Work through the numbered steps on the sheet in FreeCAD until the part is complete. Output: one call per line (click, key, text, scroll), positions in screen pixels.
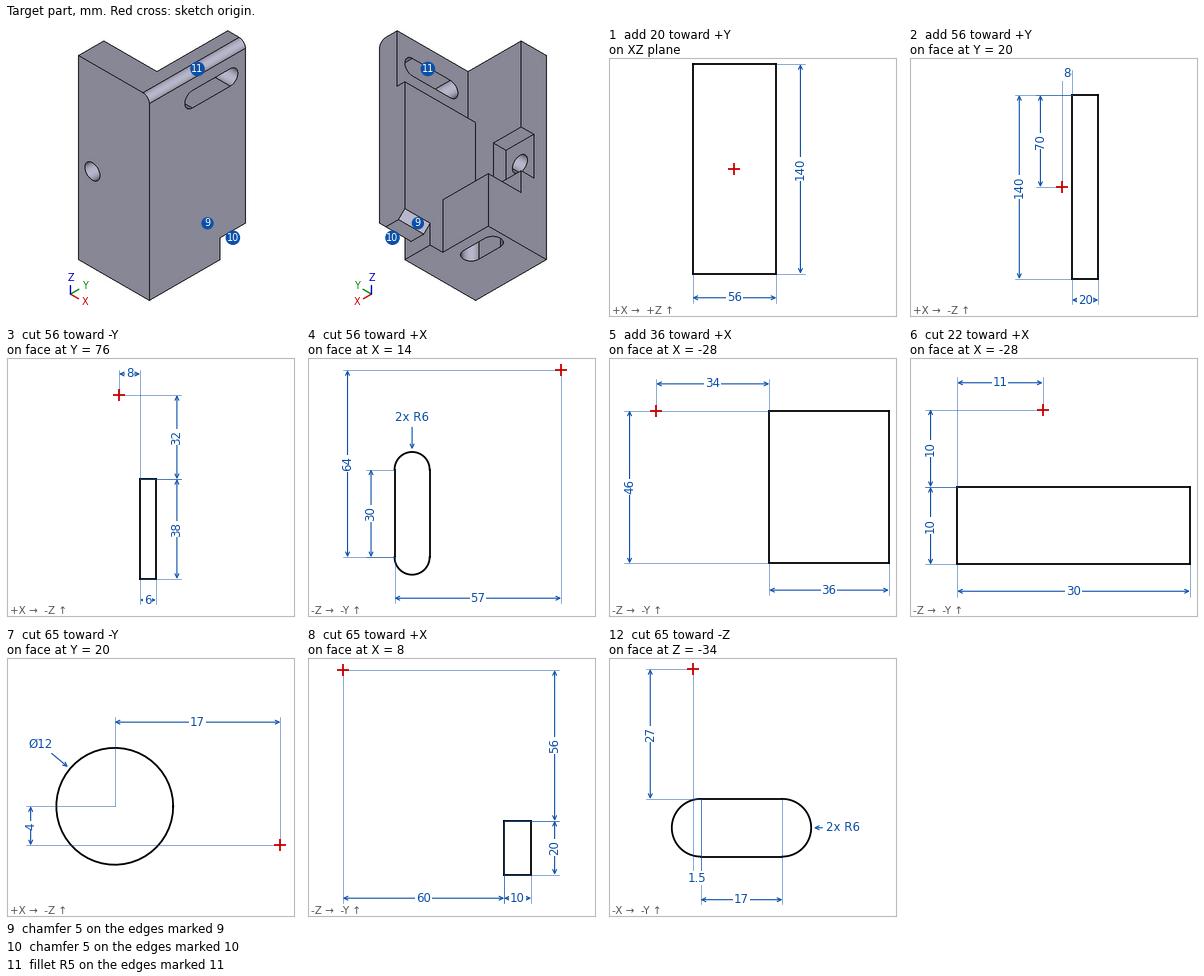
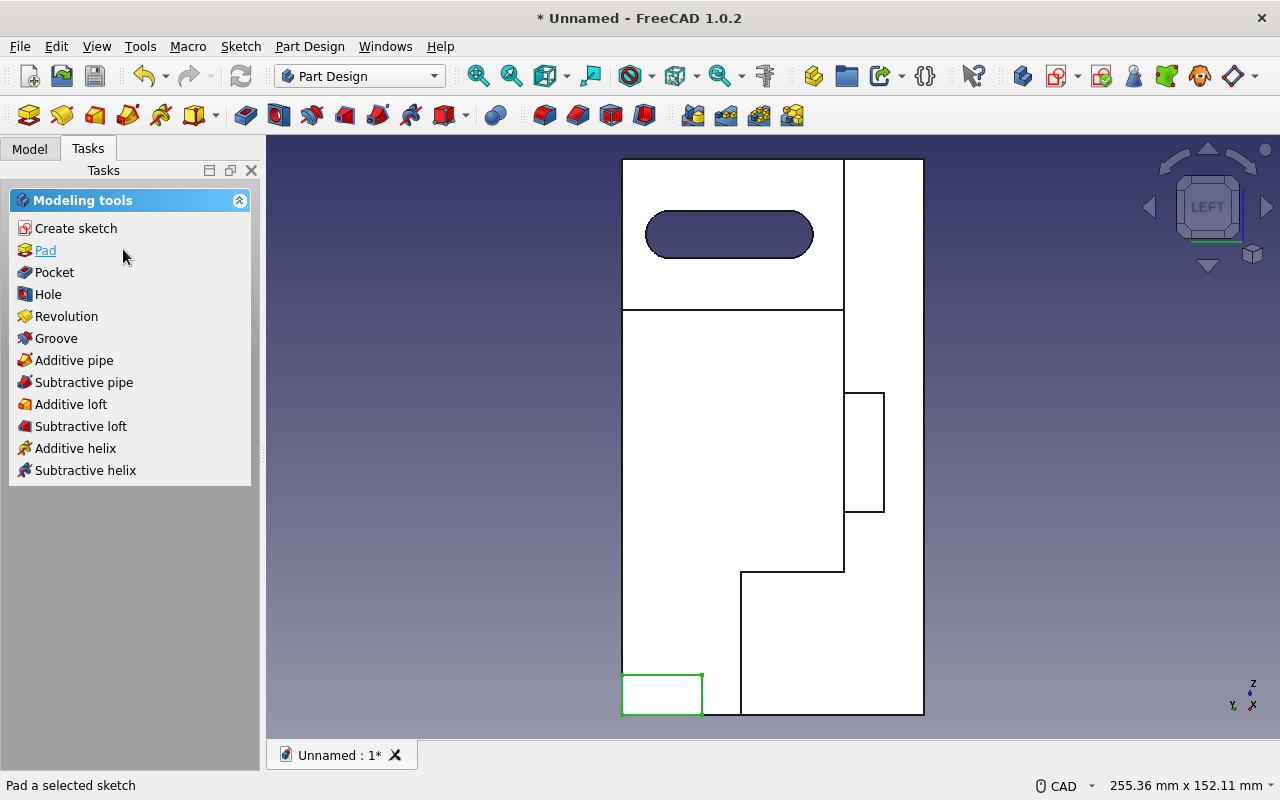
click(246, 116)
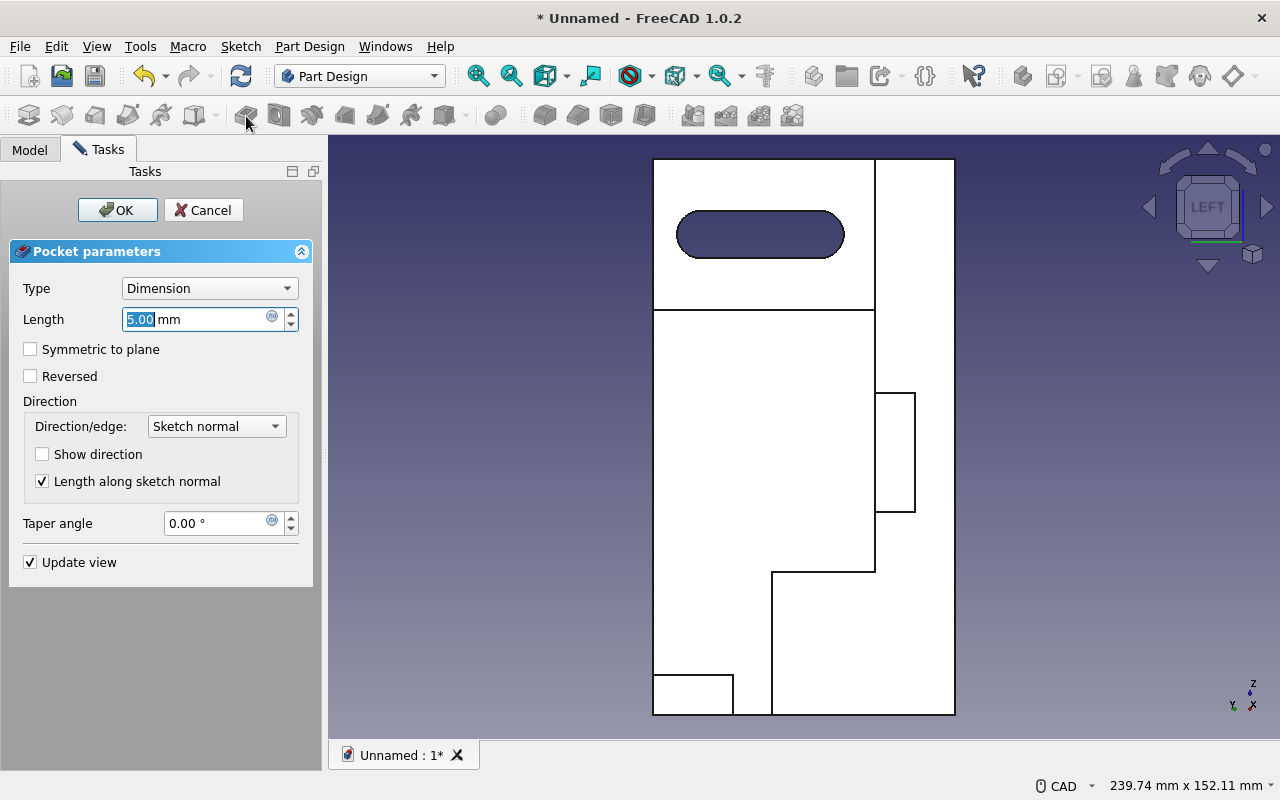
text(65)
key(Tab)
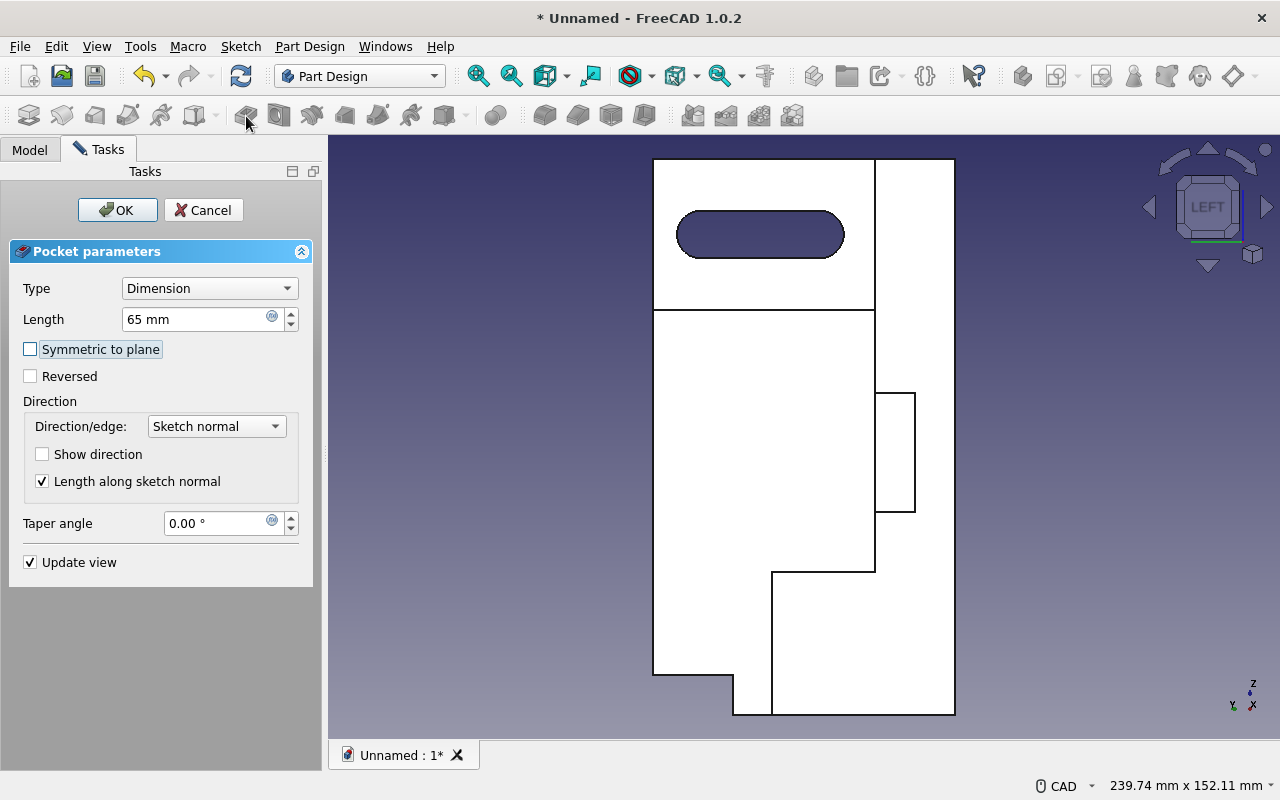
click(118, 210)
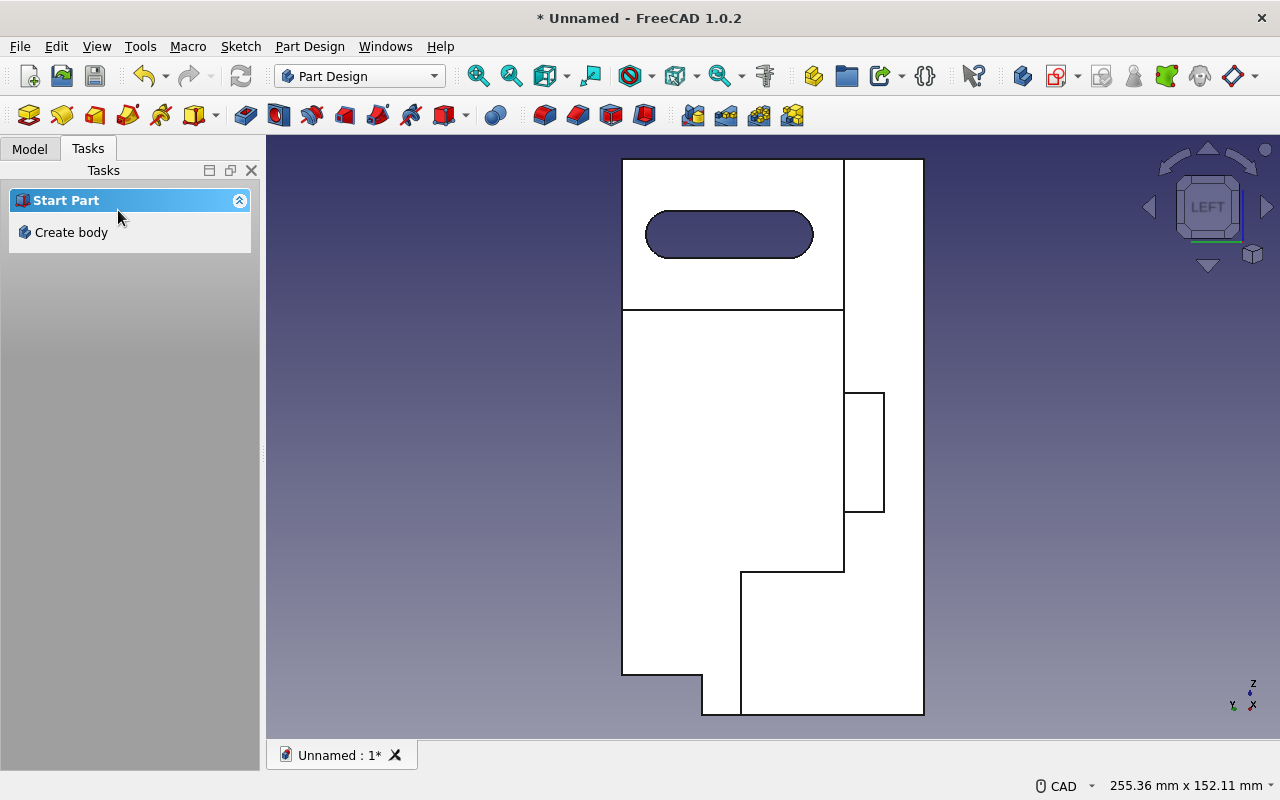
click(662, 674)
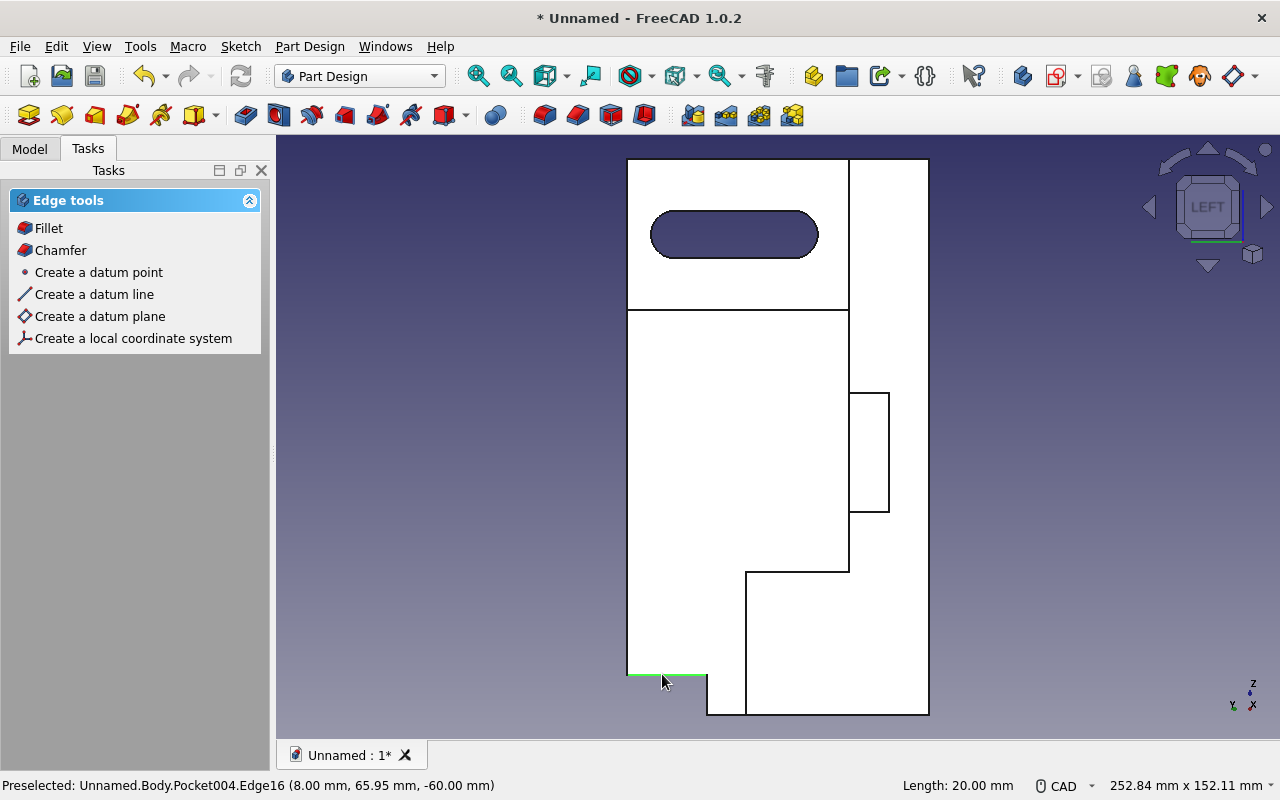
click(578, 116)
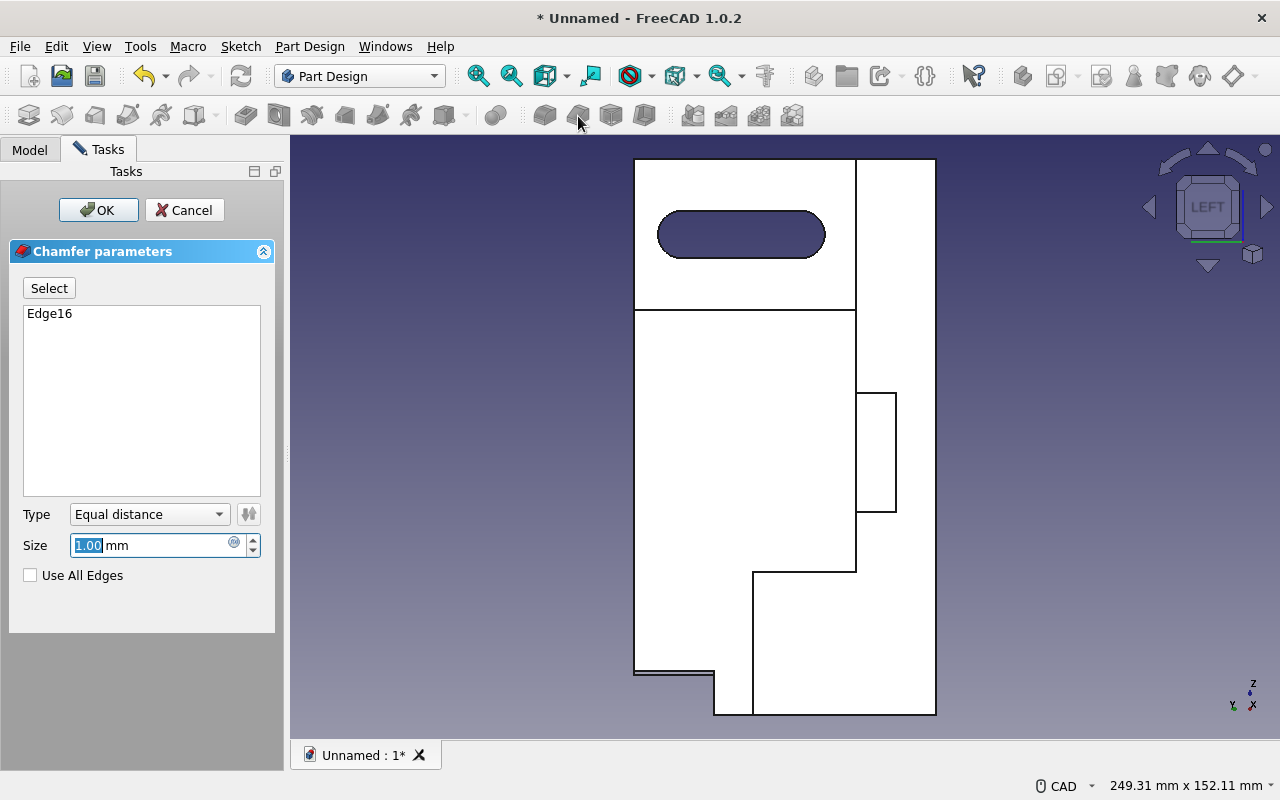
text(5)
key(Tab)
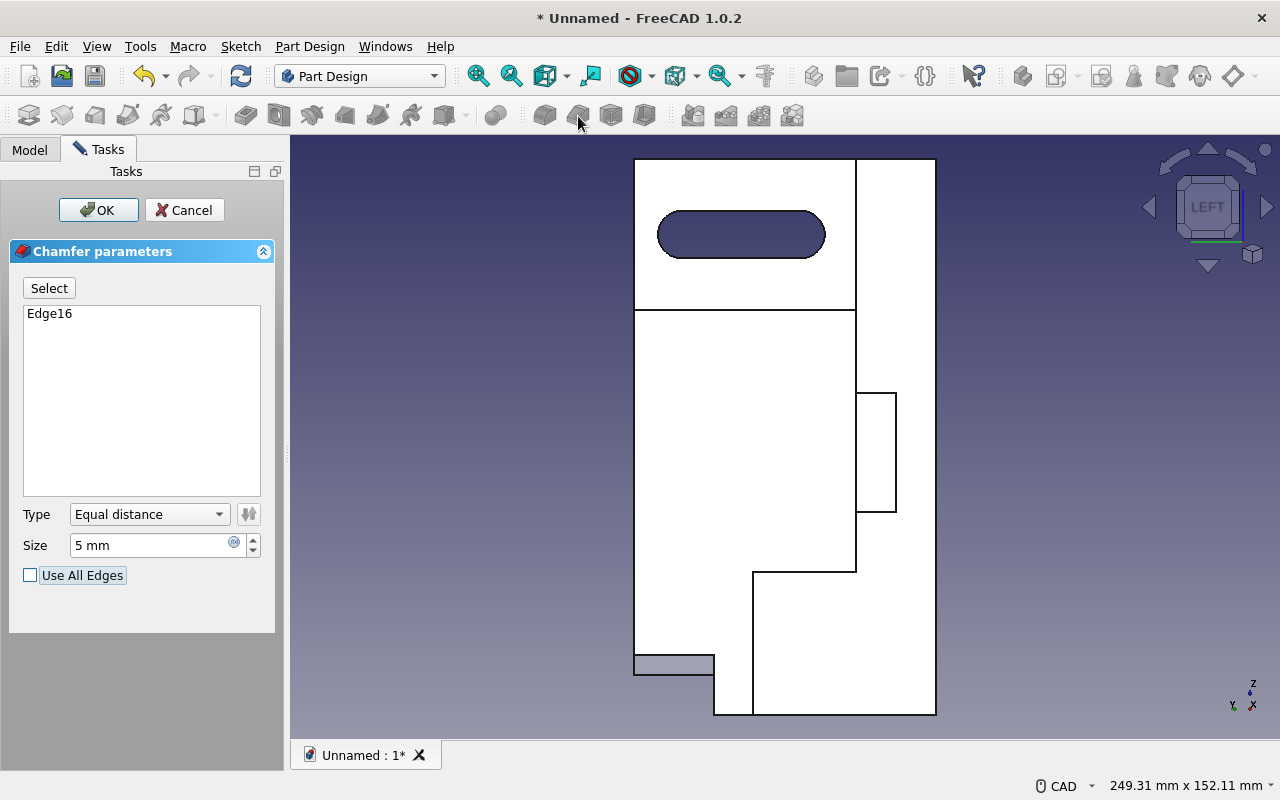
click(99, 210)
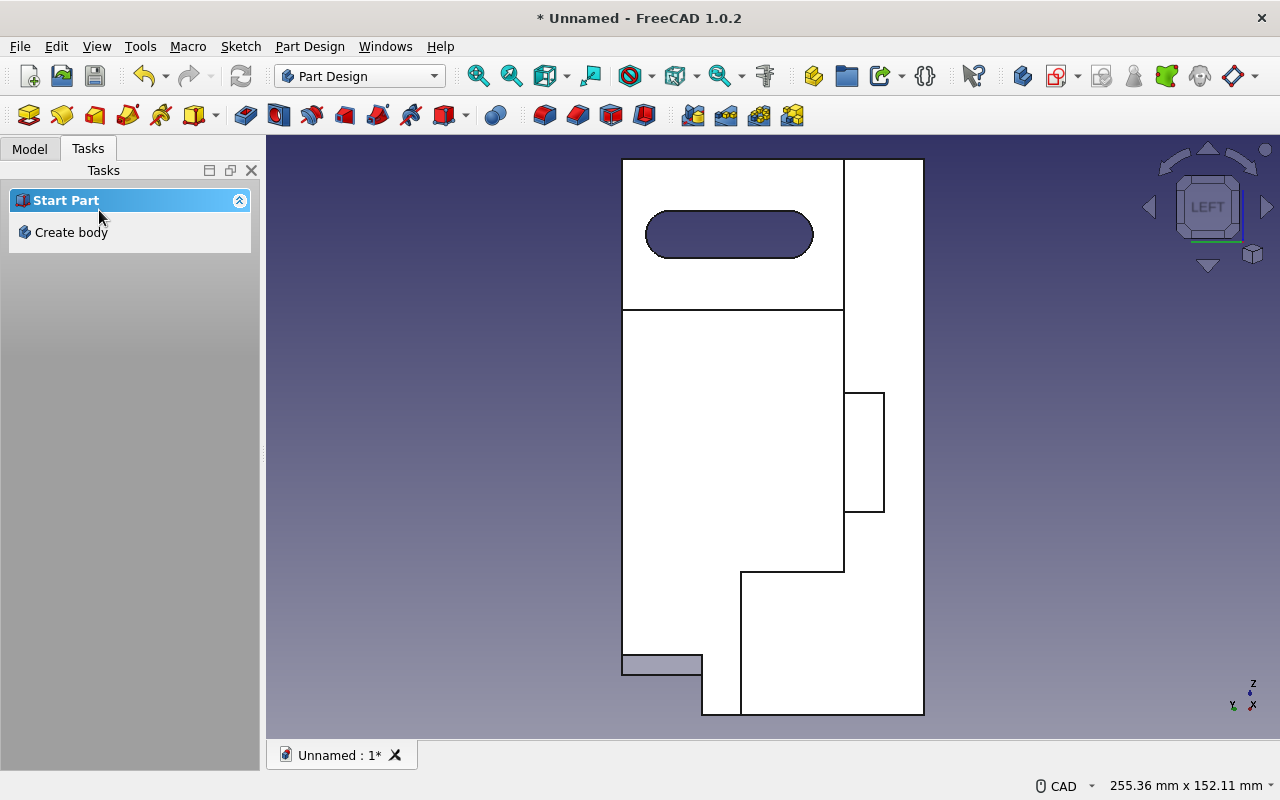
key(0)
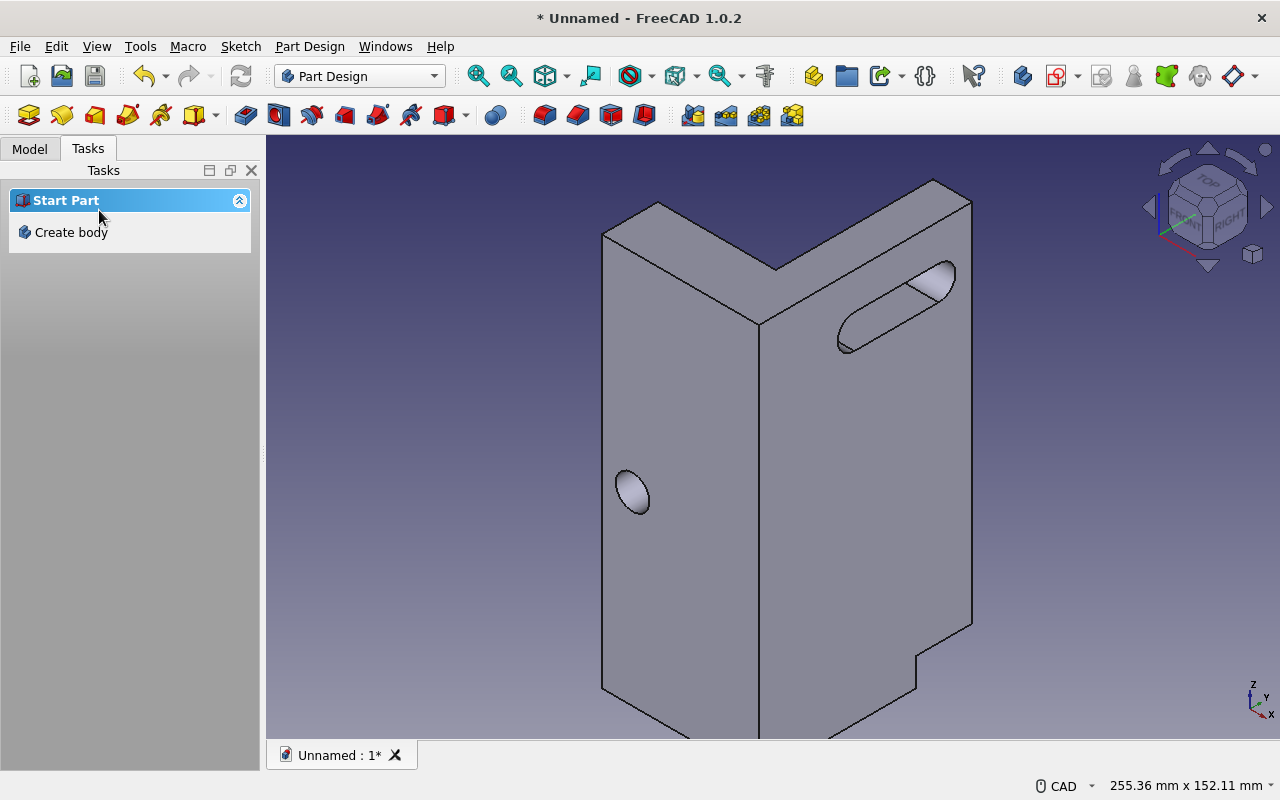
click(479, 76)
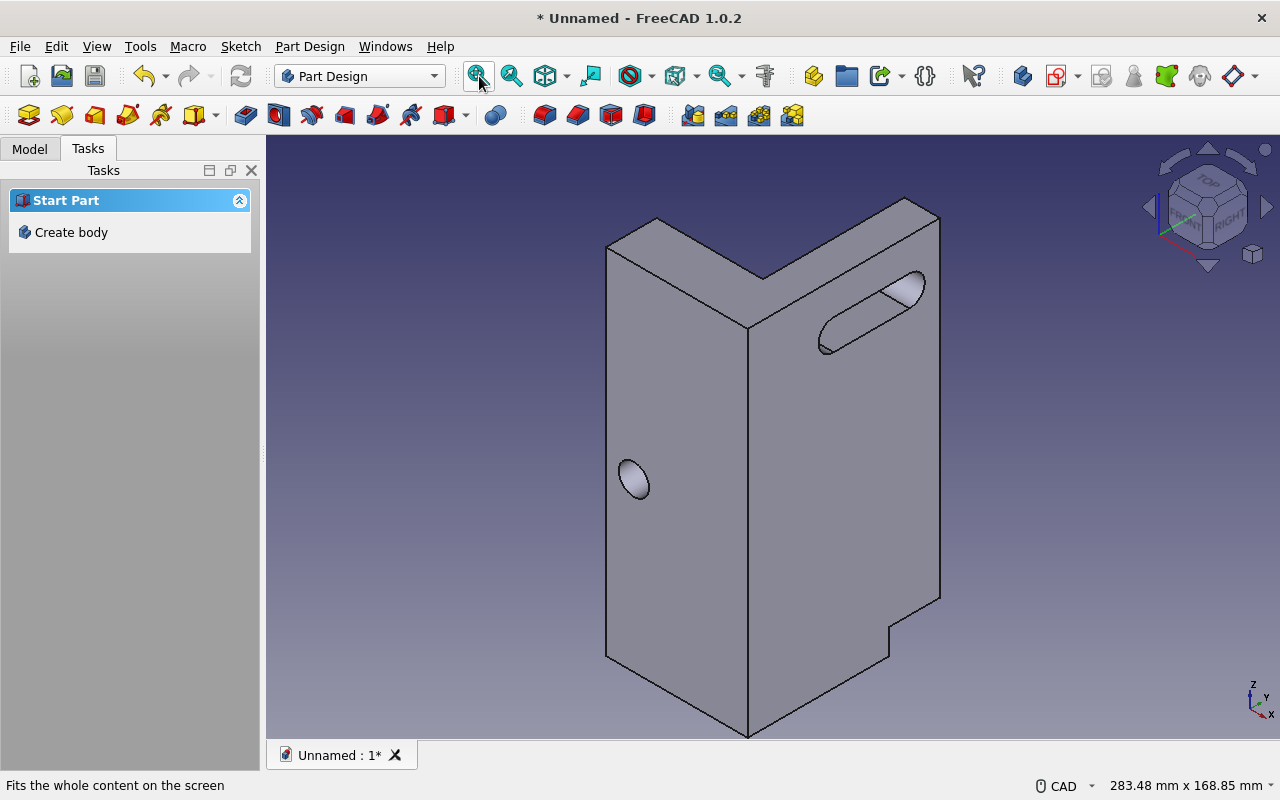
key(2)